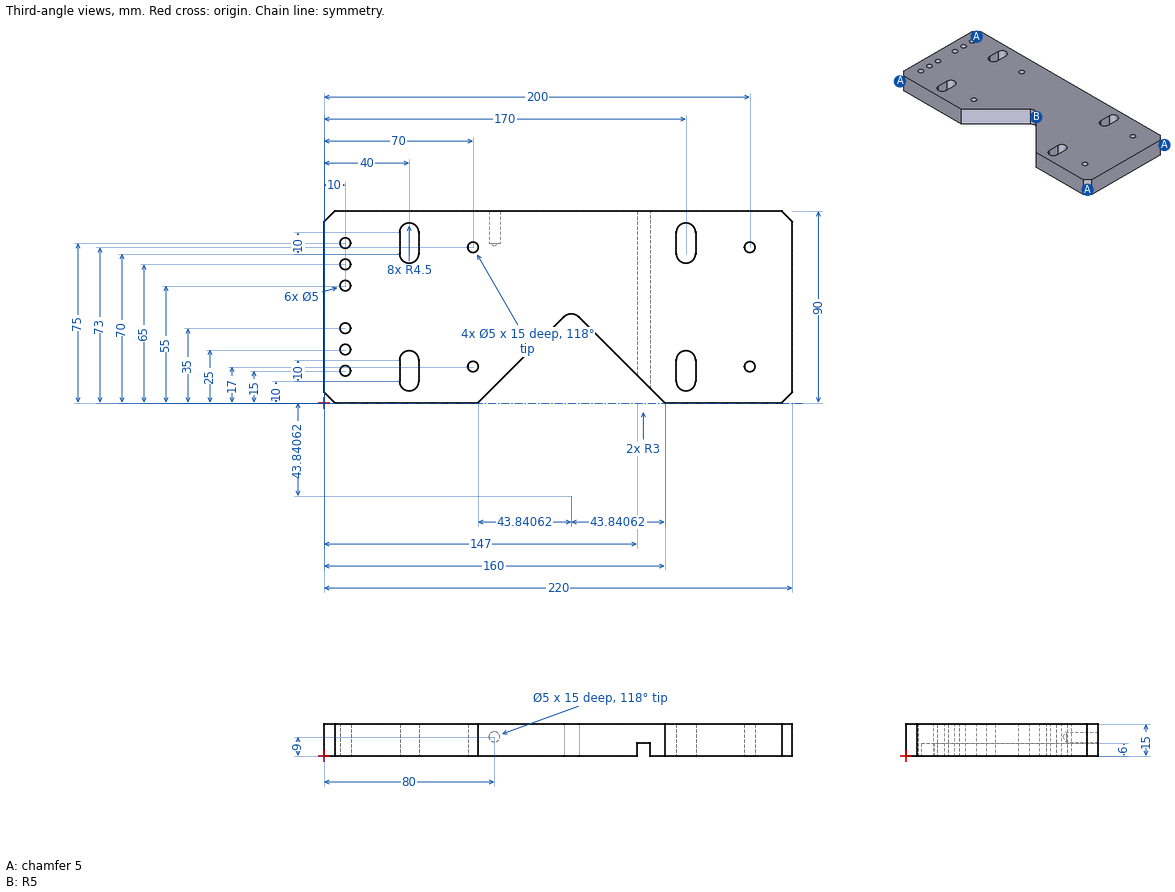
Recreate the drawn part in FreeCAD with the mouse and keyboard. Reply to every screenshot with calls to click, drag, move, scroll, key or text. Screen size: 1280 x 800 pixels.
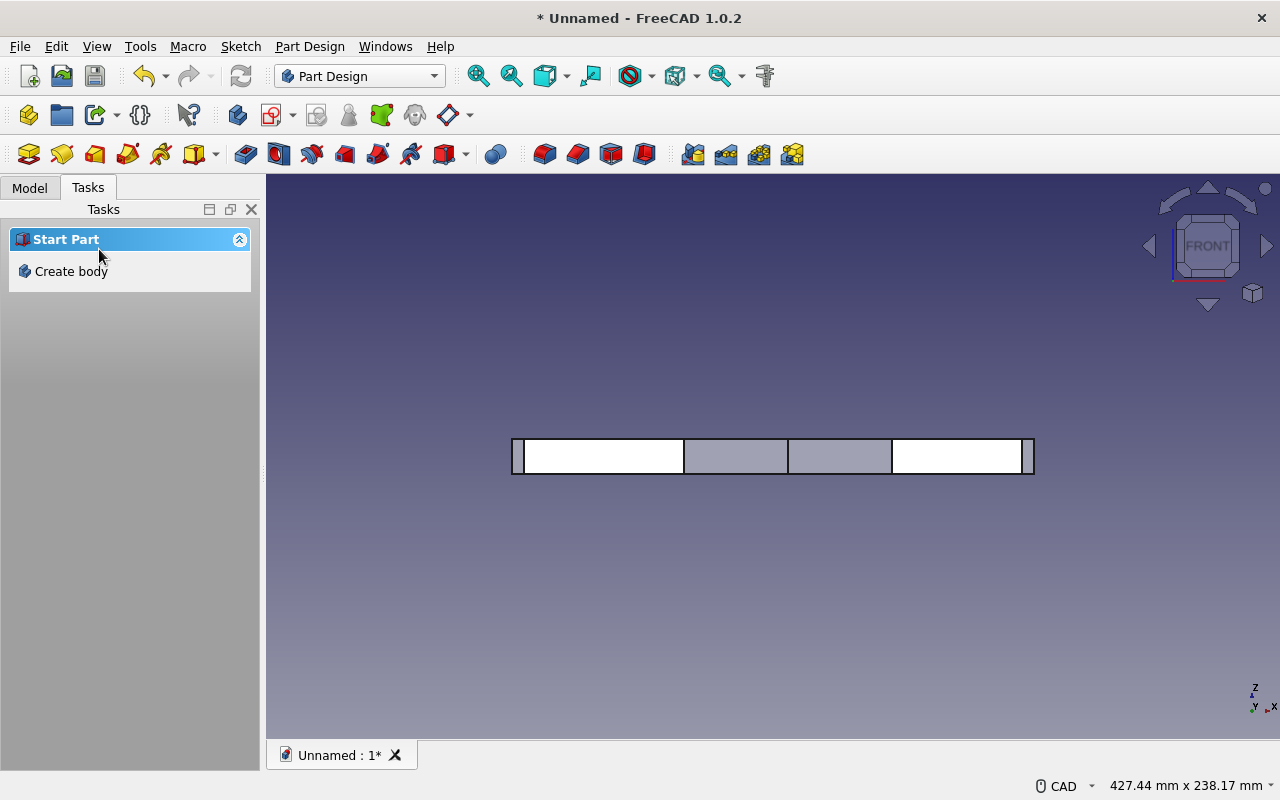
key(3)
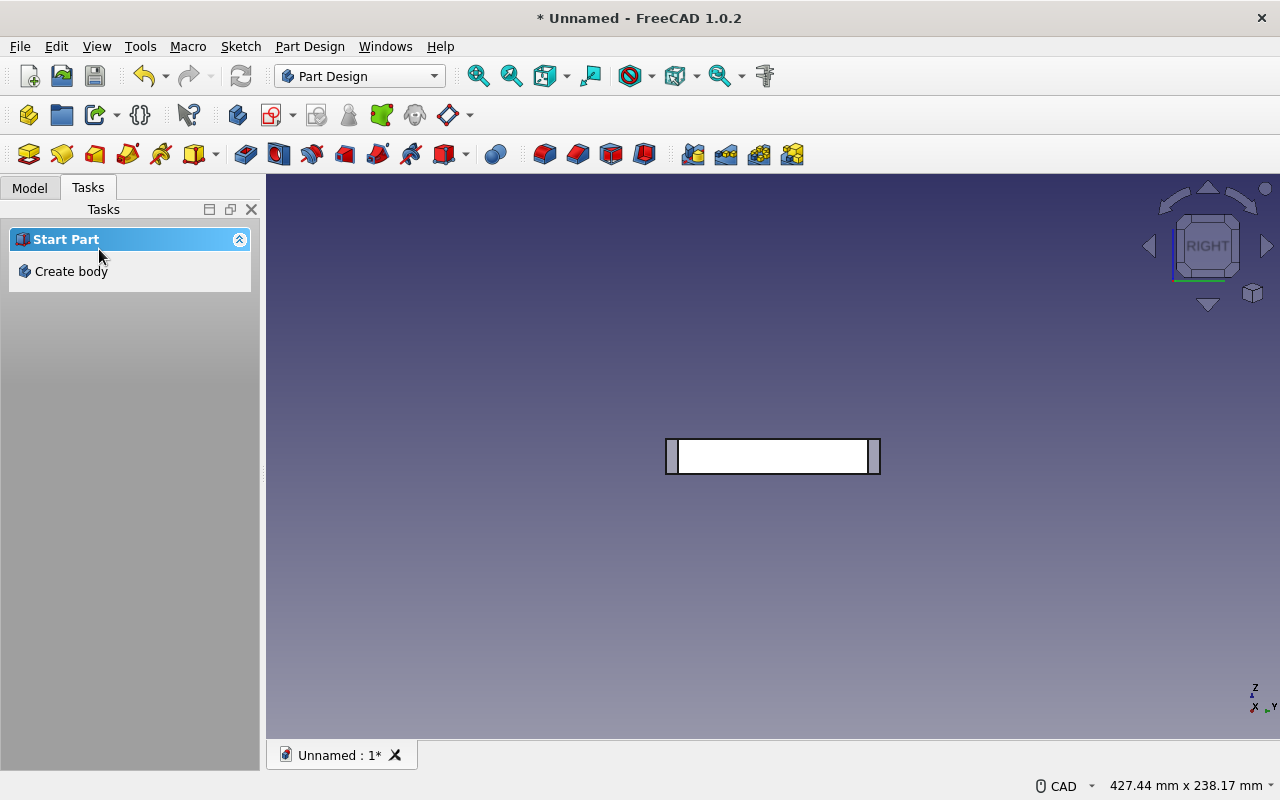
click(479, 76)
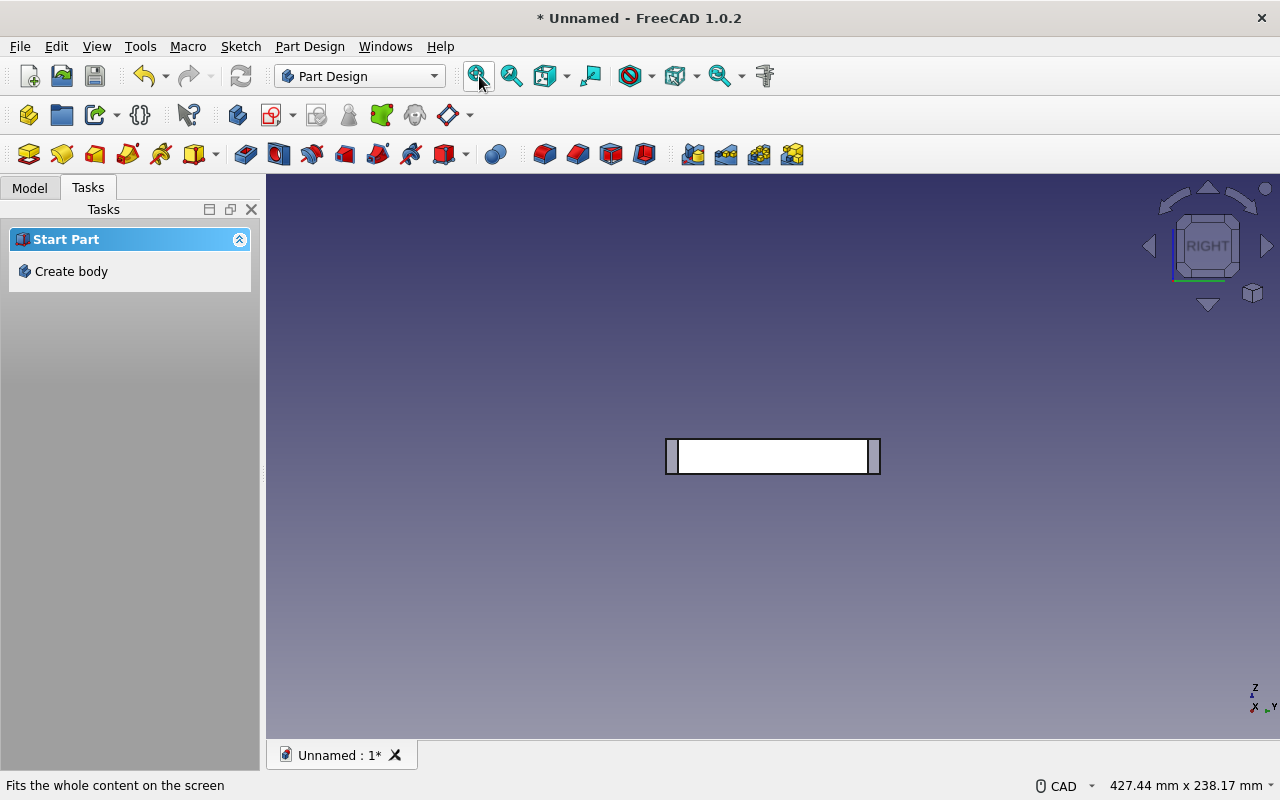
key(5)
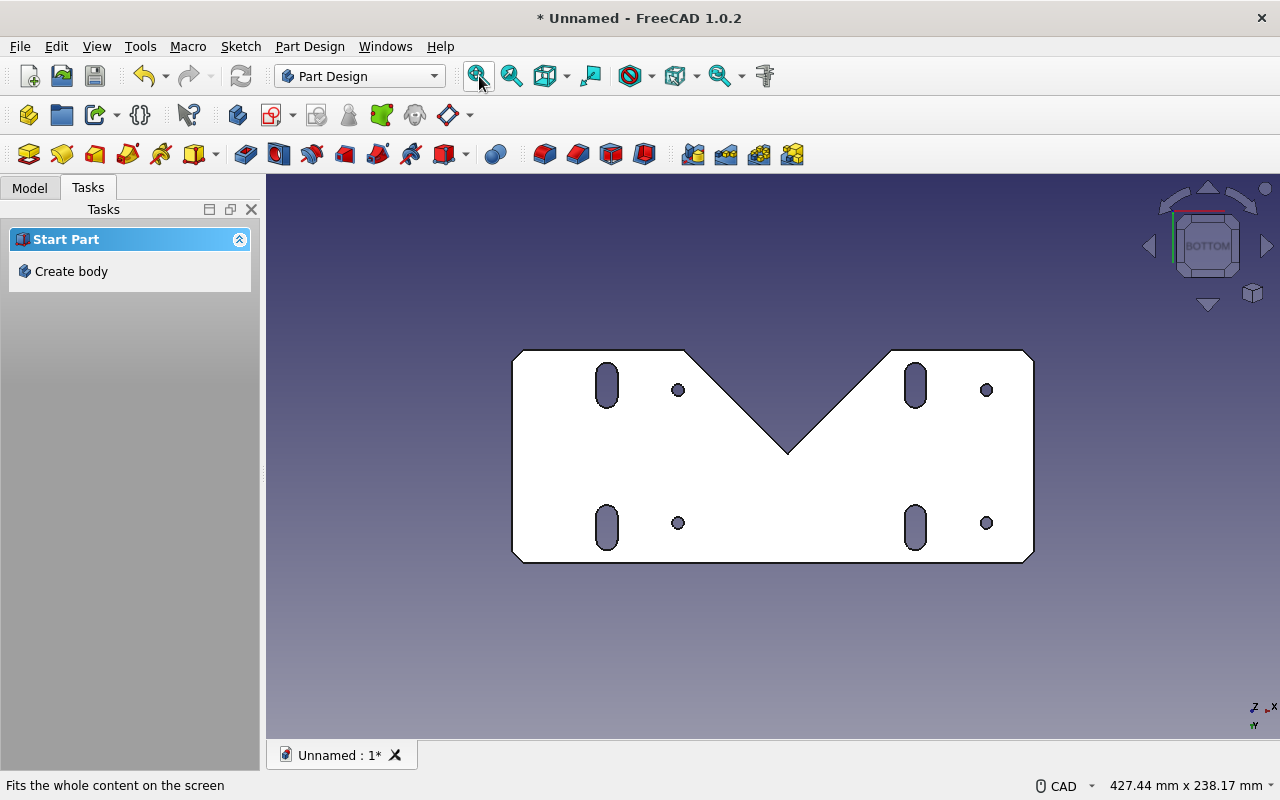
key(4)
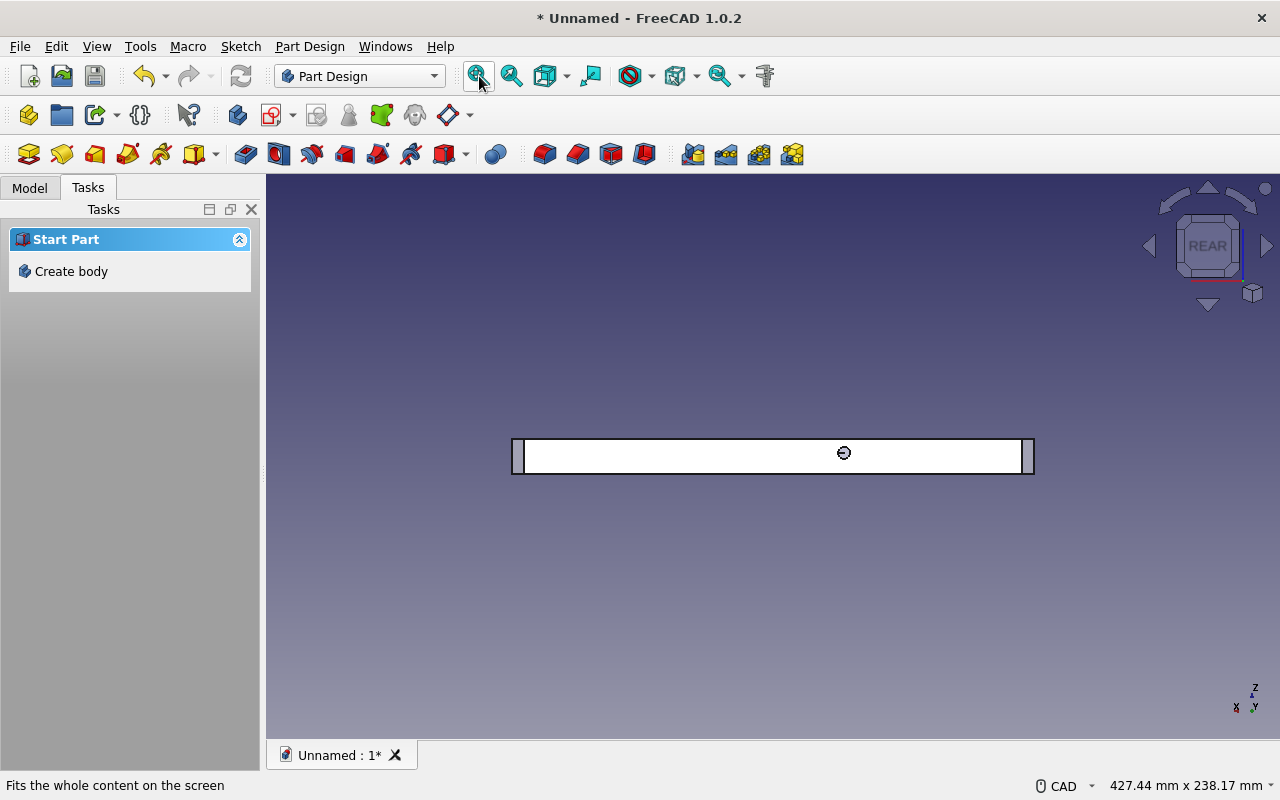
key(6)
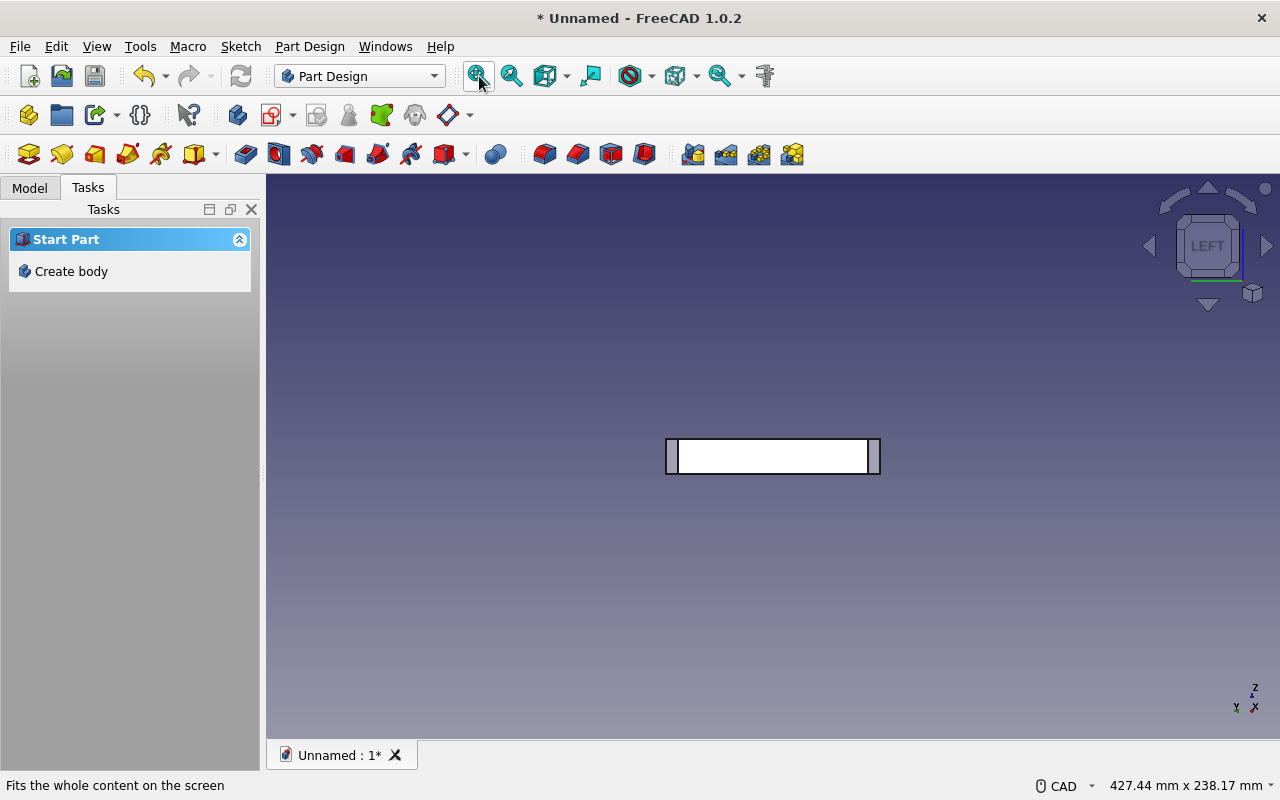
click(479, 76)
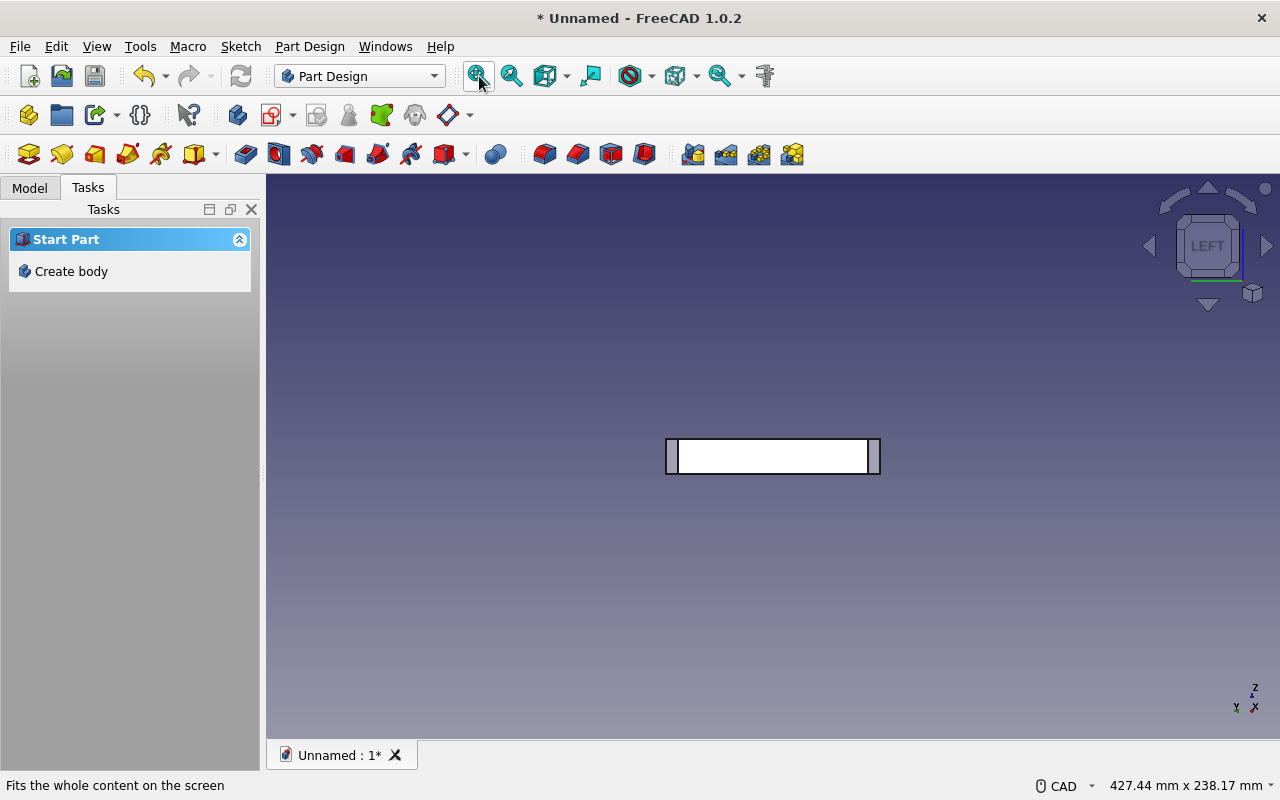
key(v)
key(3)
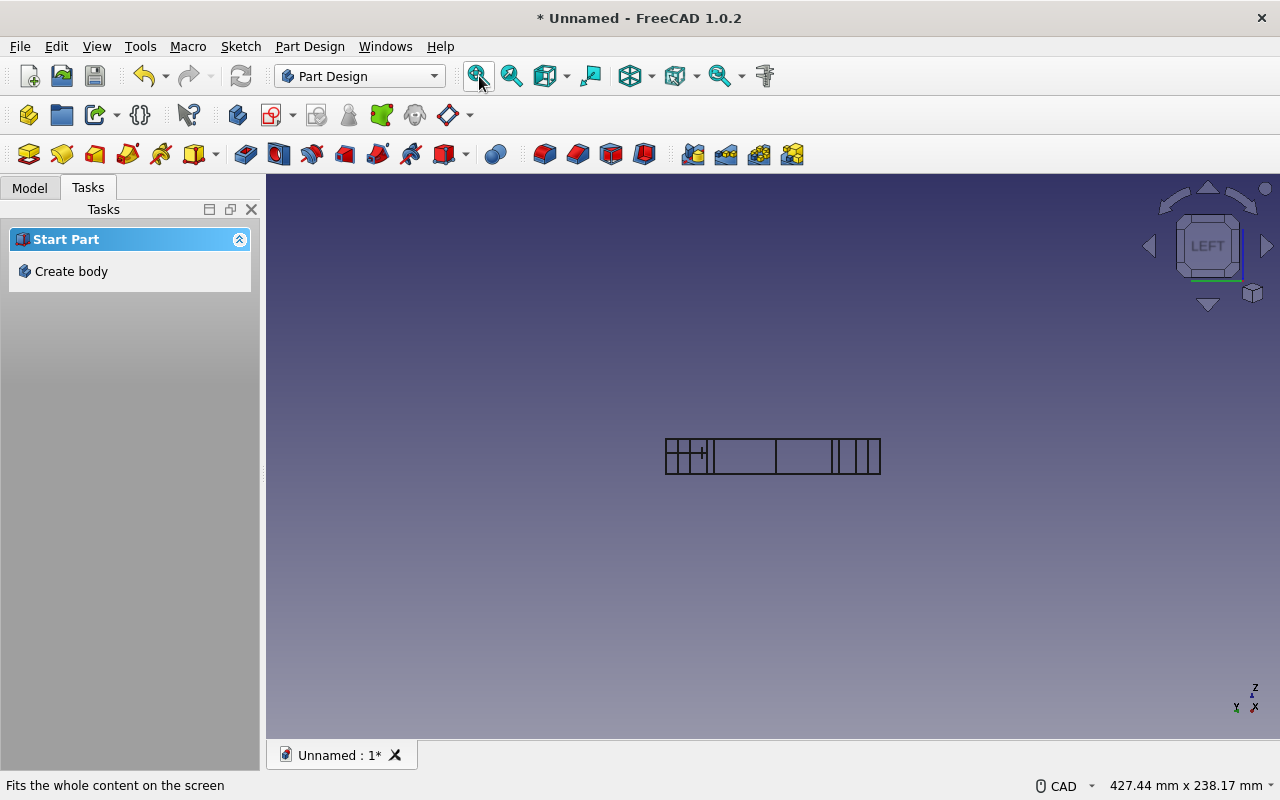
key(0)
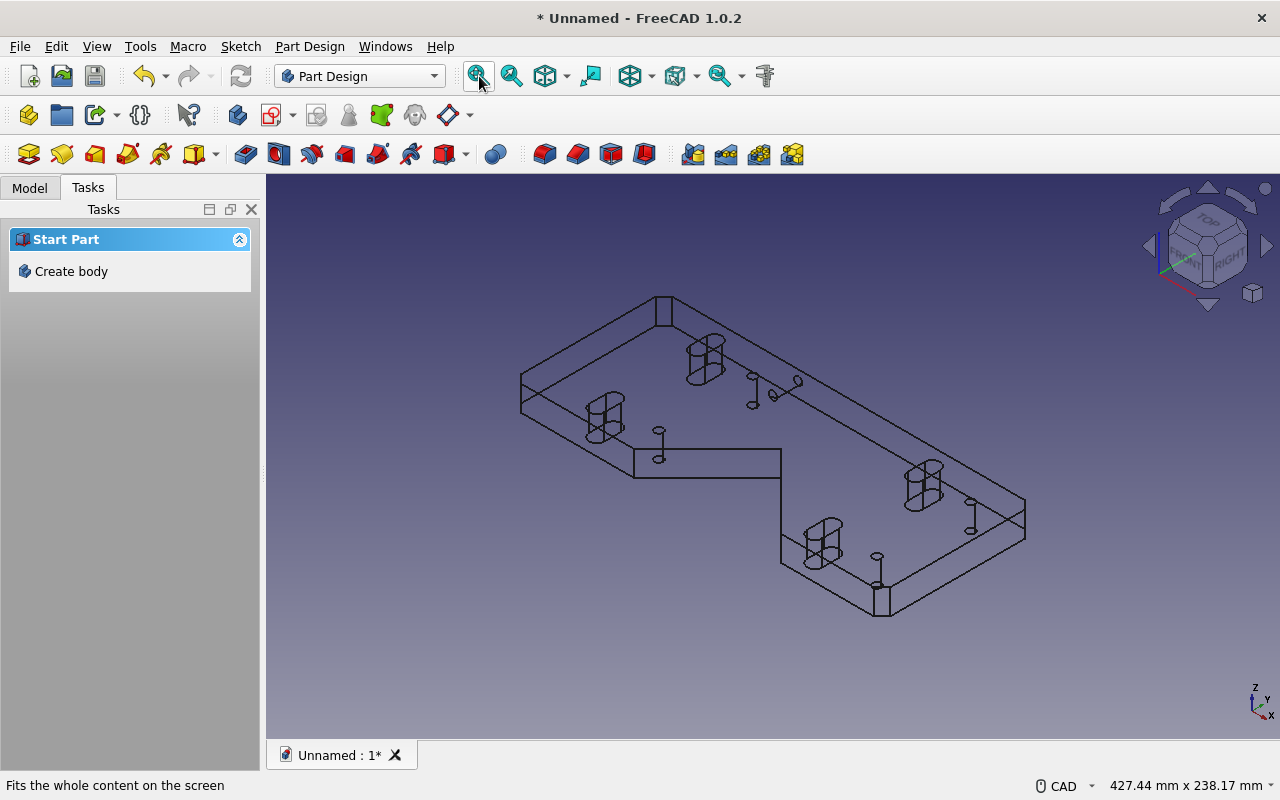
key(2)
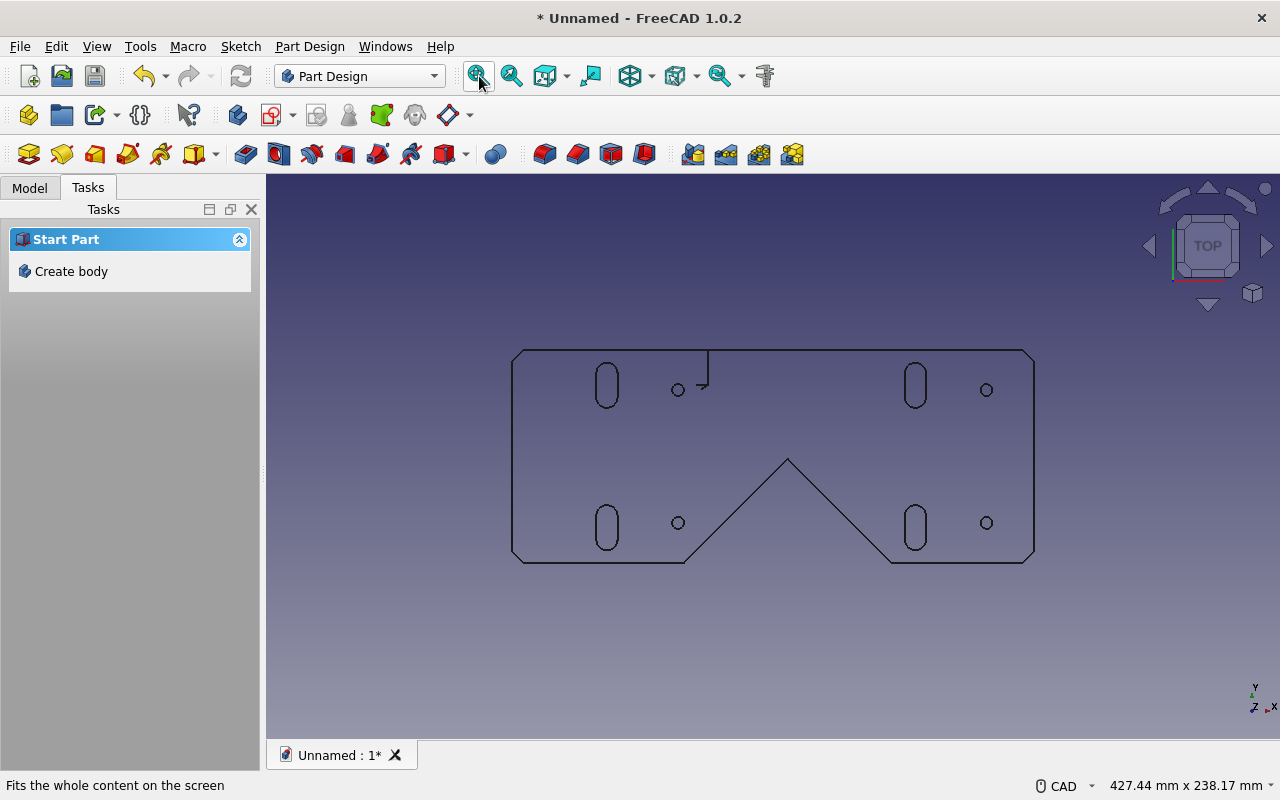
key(1)